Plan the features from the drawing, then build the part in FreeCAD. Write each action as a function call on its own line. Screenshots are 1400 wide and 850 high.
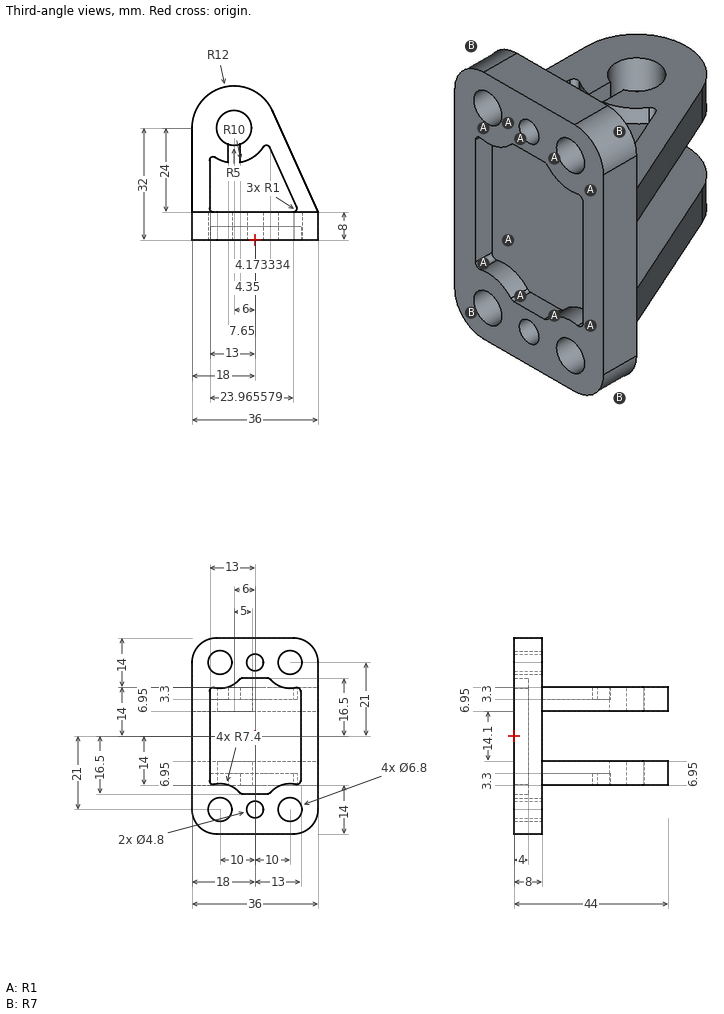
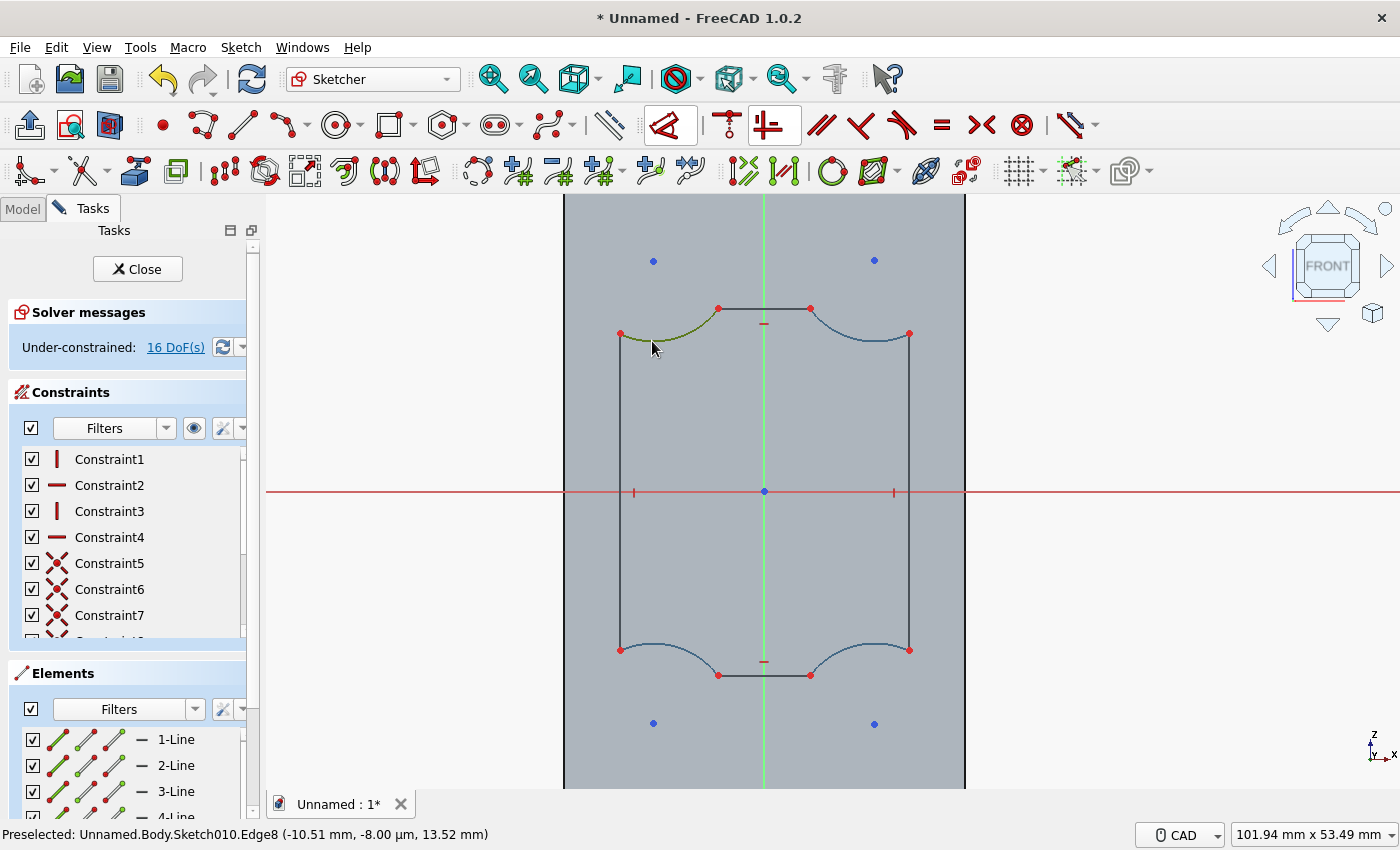
key(e)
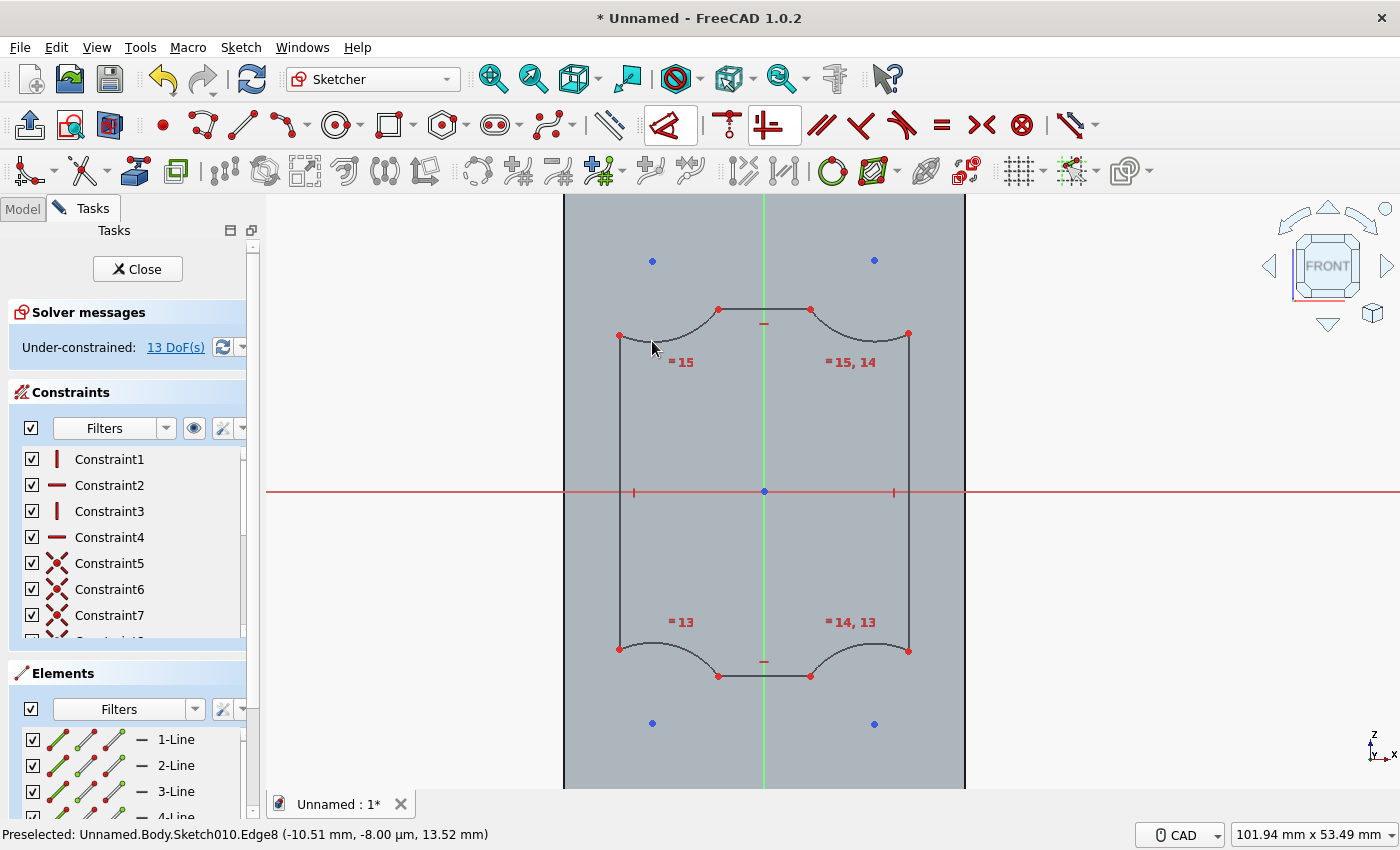
click(694, 654)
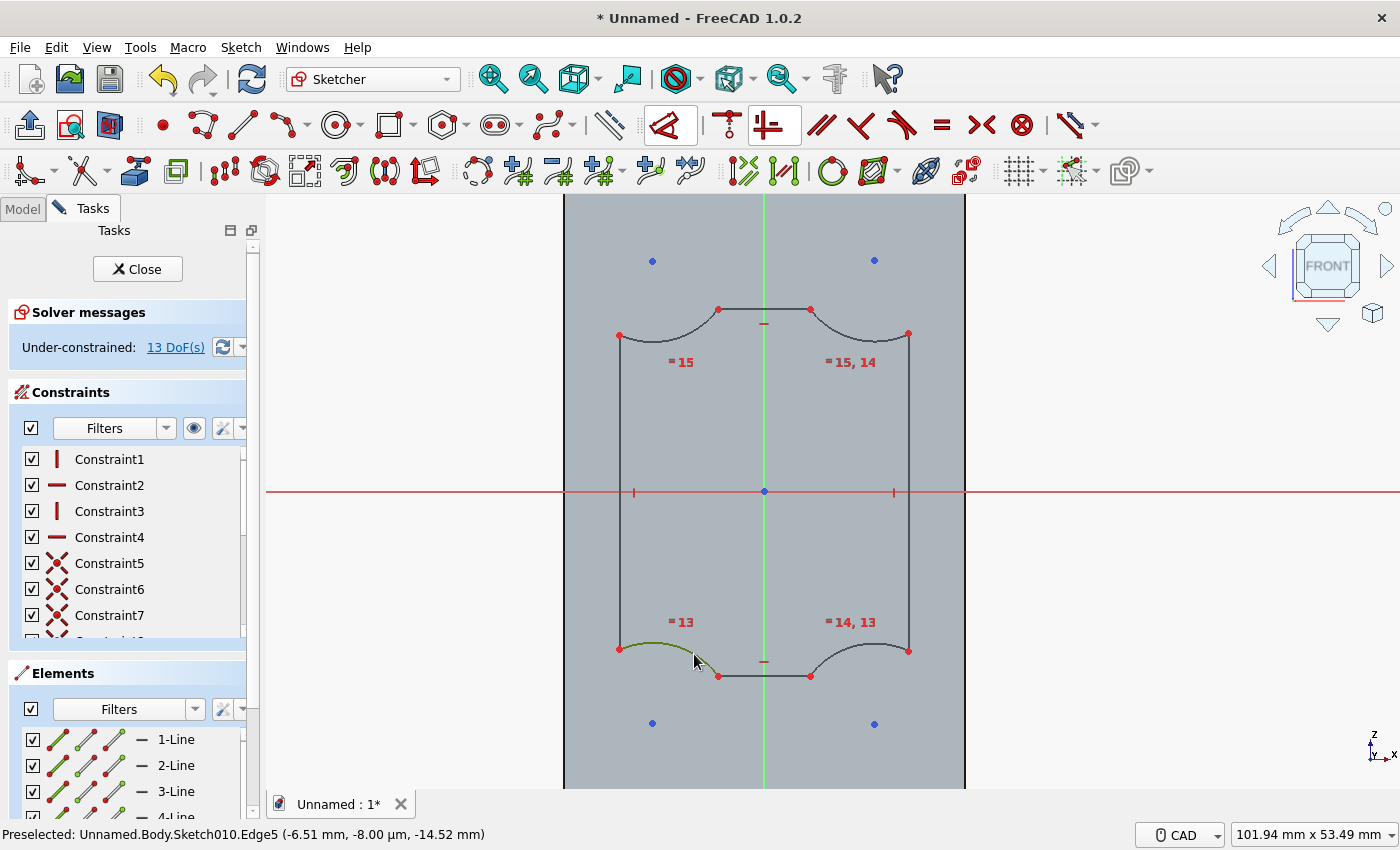
click(692, 126)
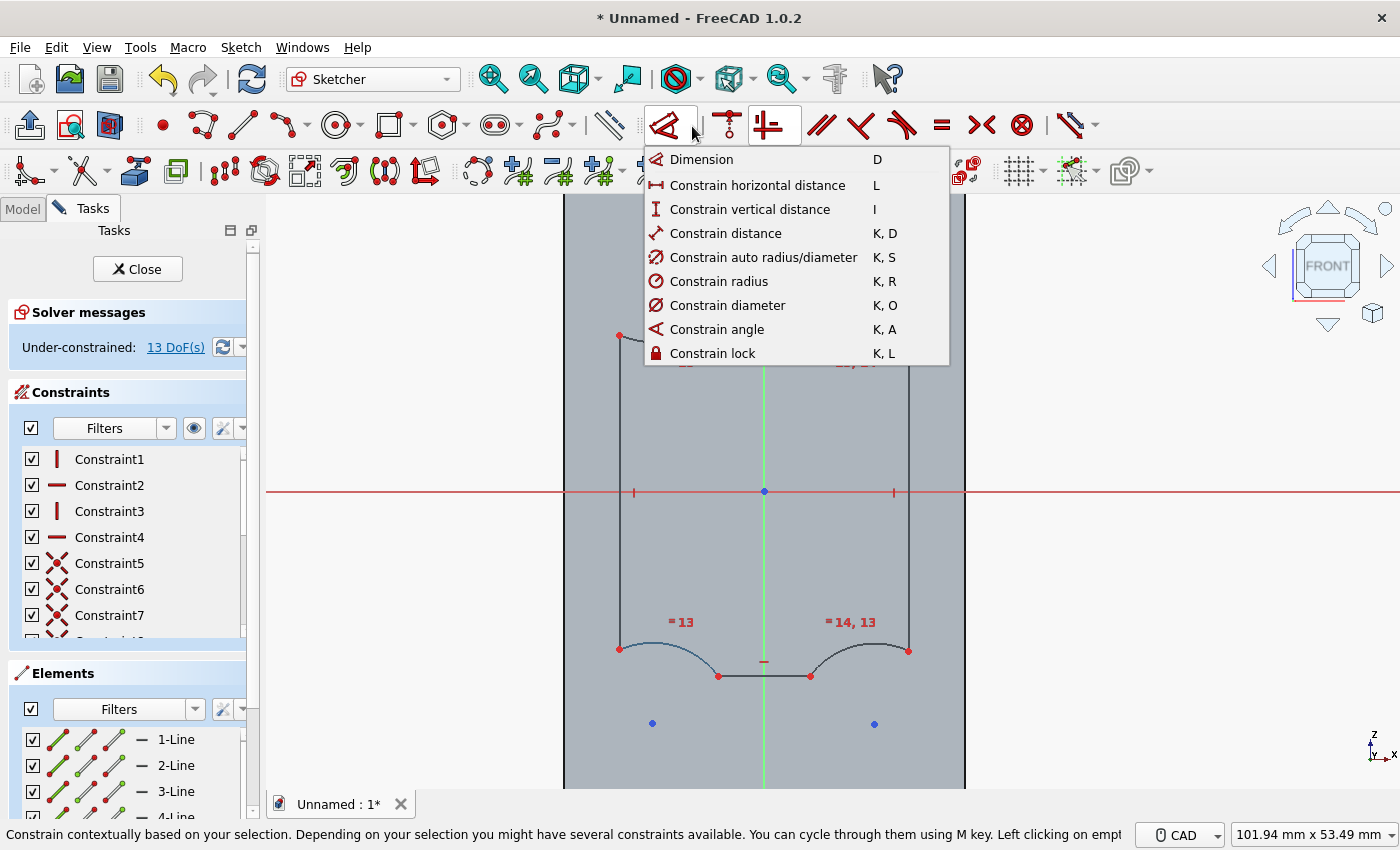
click(797, 281)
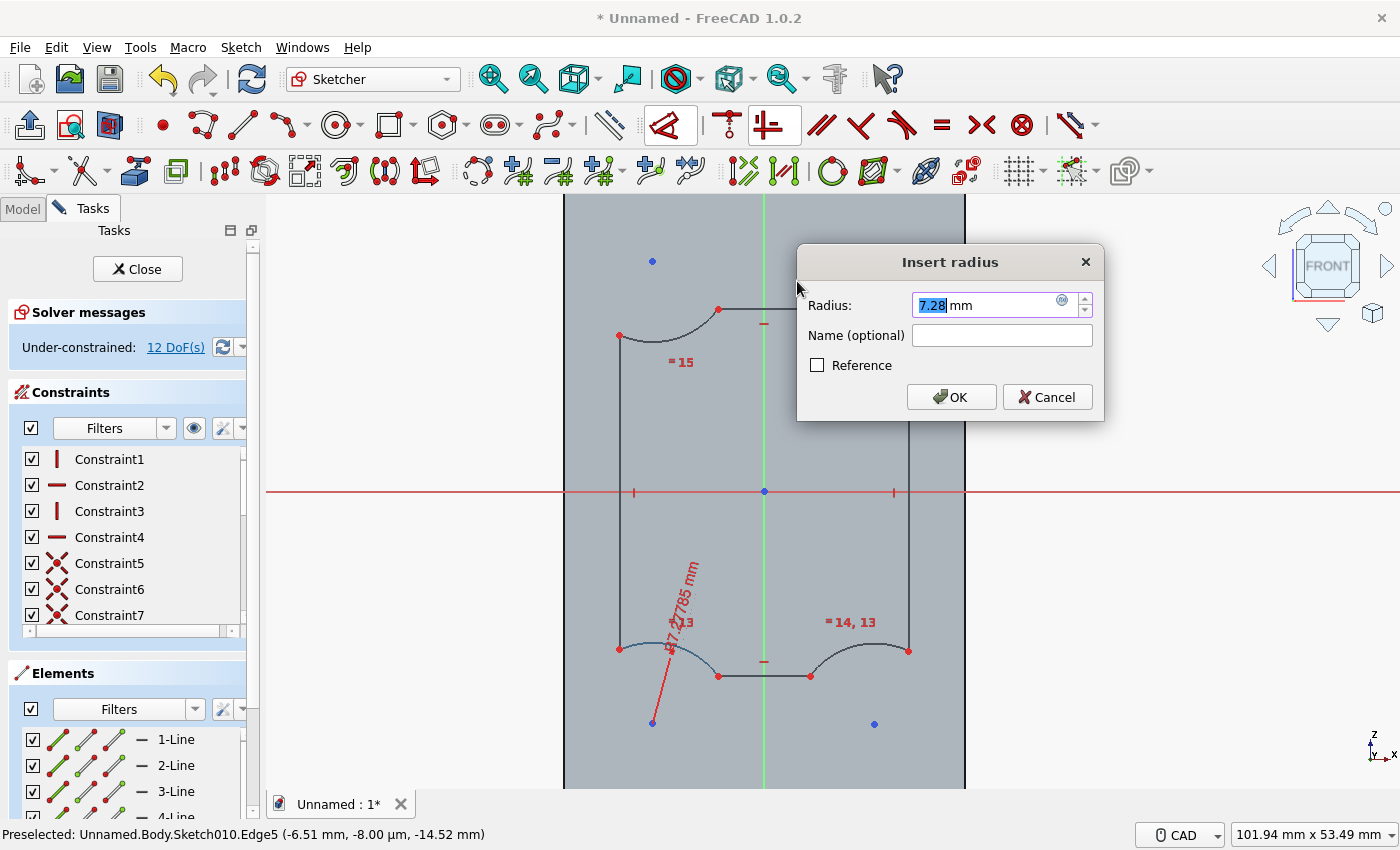
text(7.4)
key(Return)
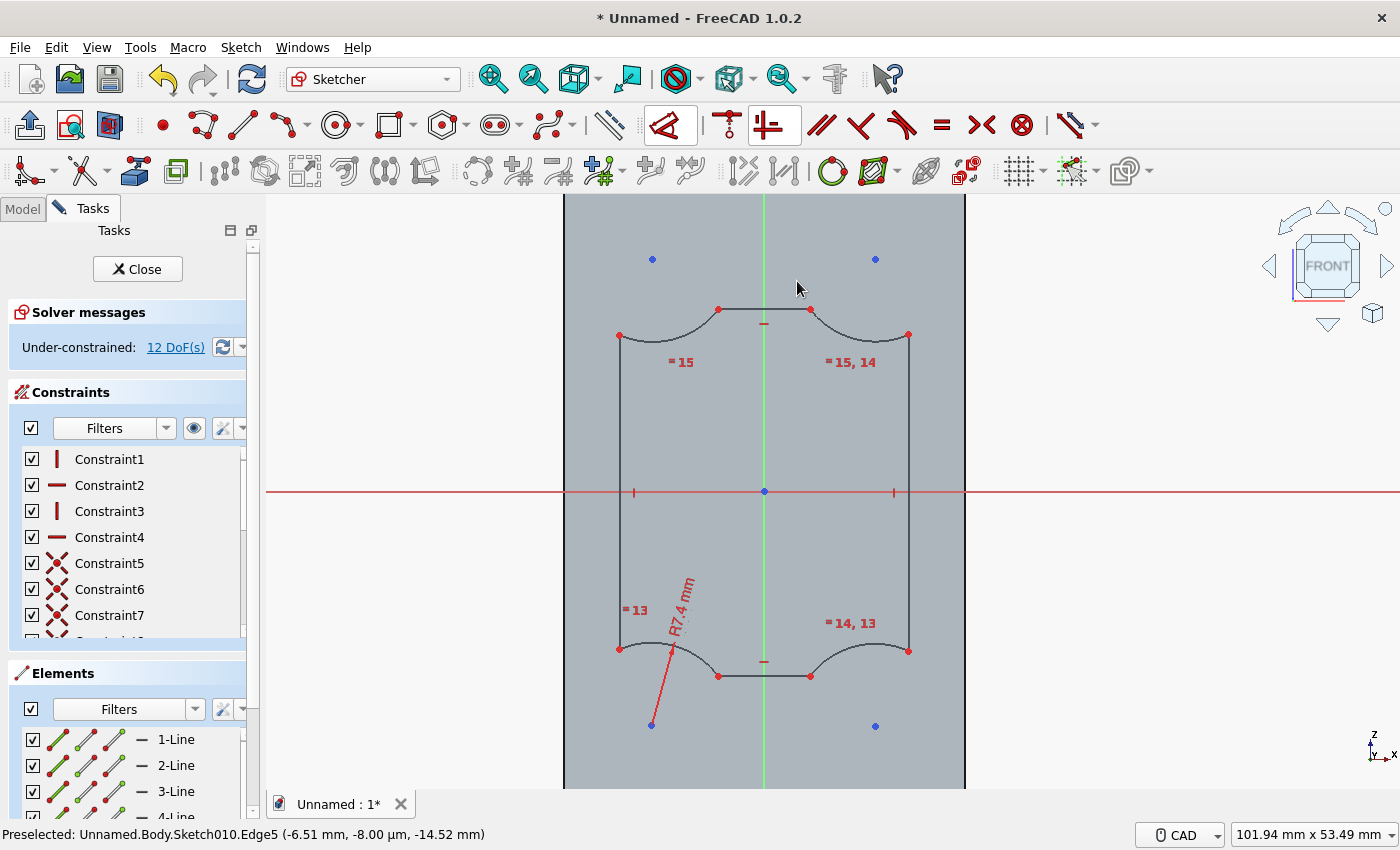
click(620, 335)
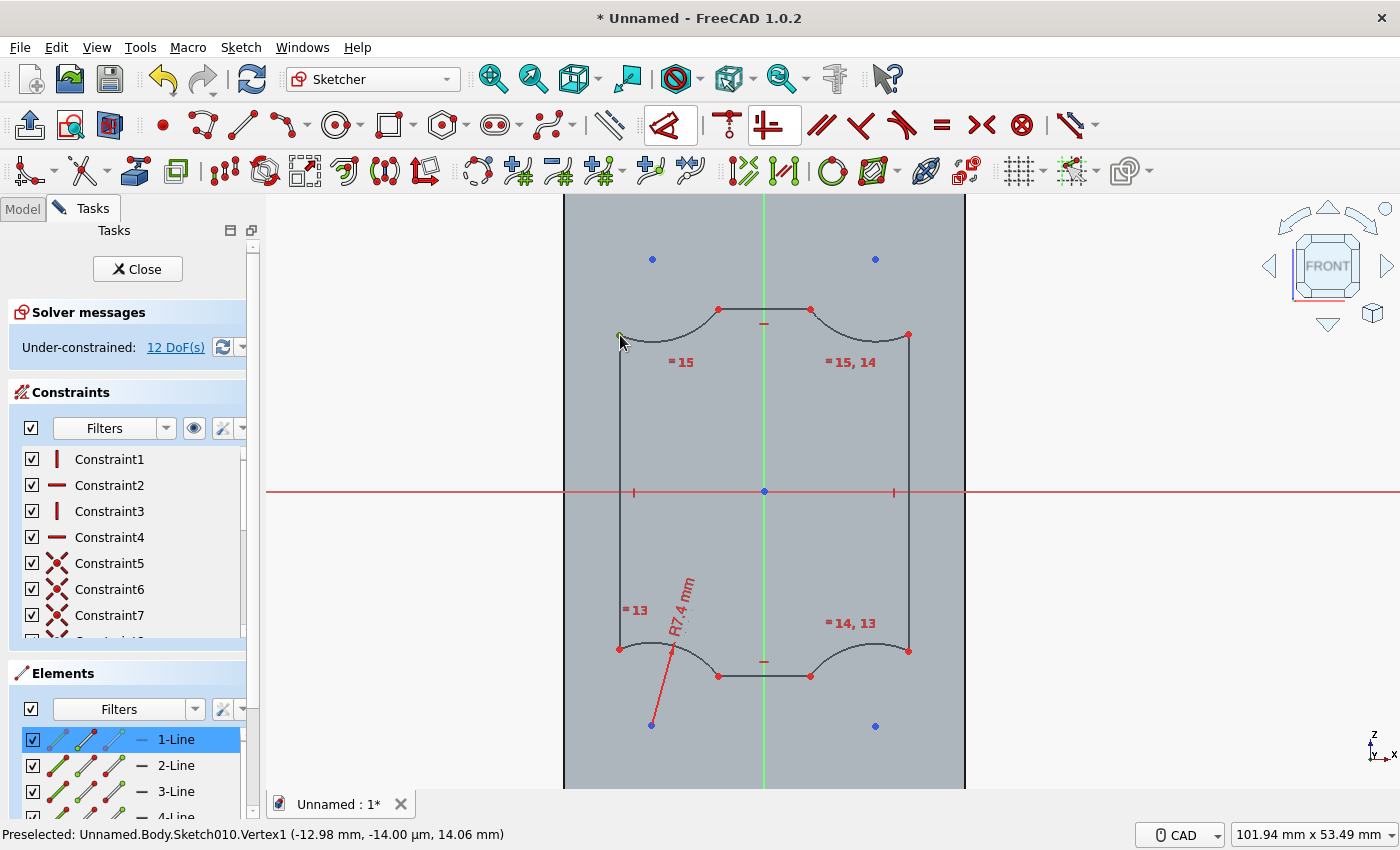
key(l)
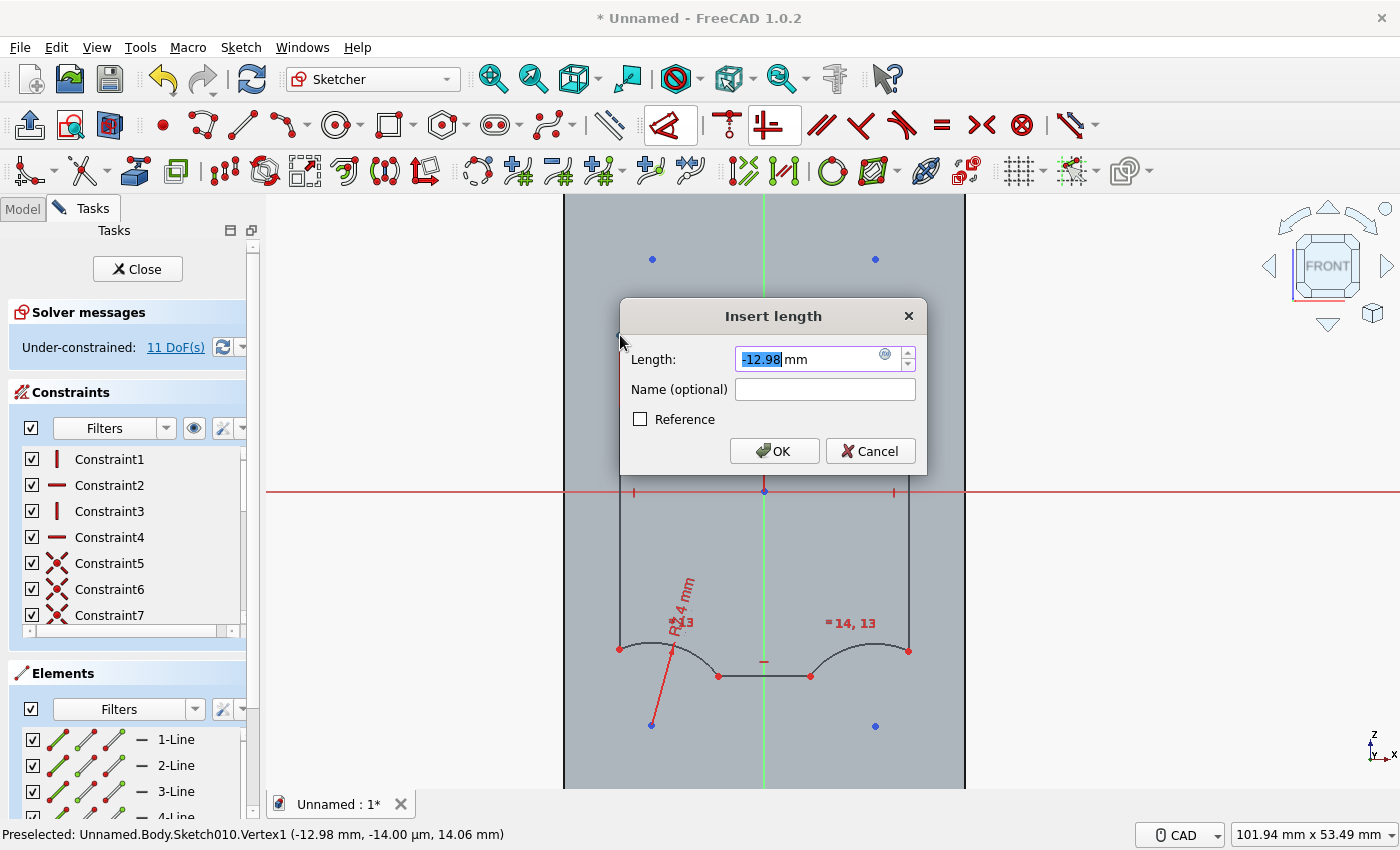
text(-13)
key(Return)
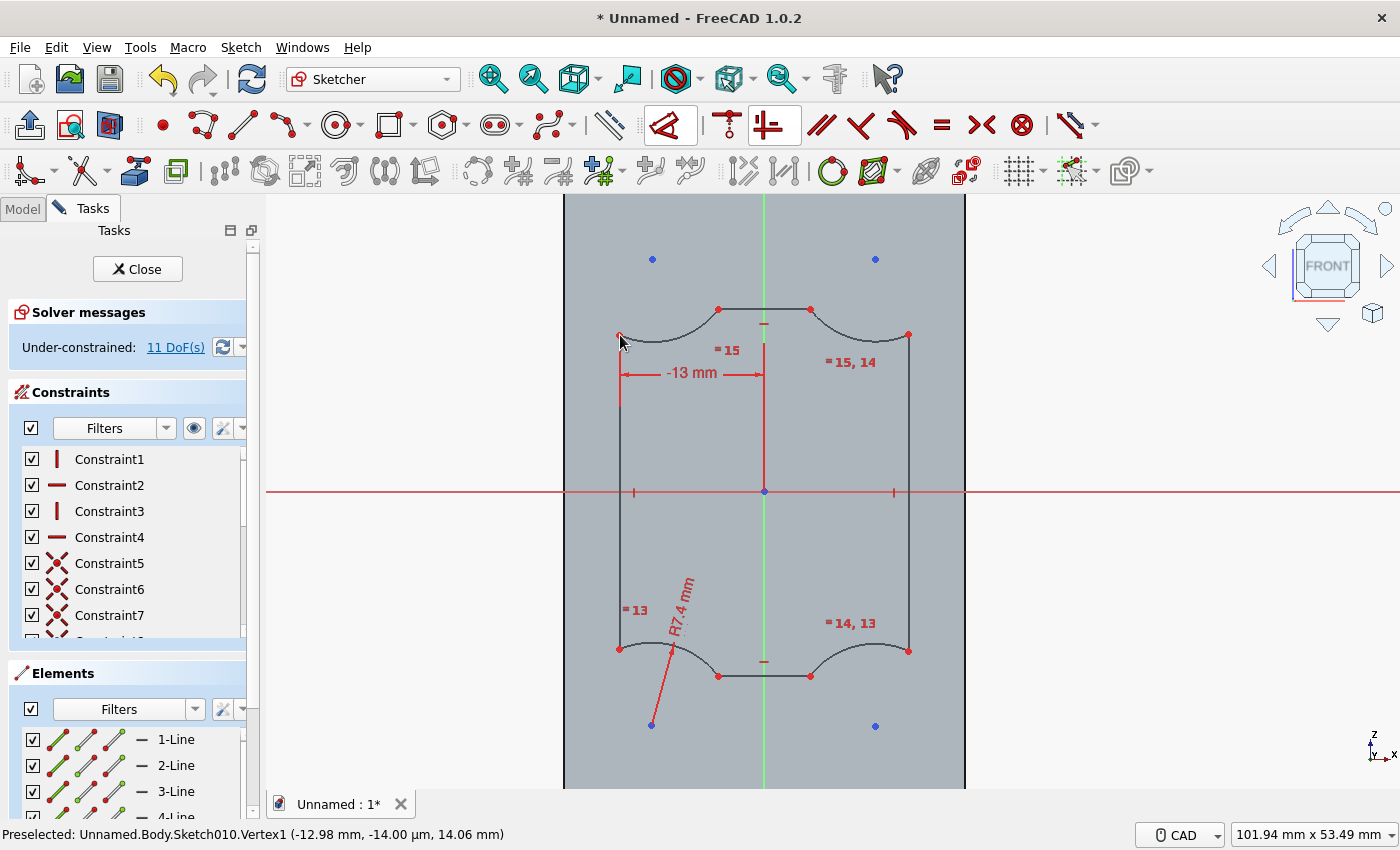
click(909, 651)